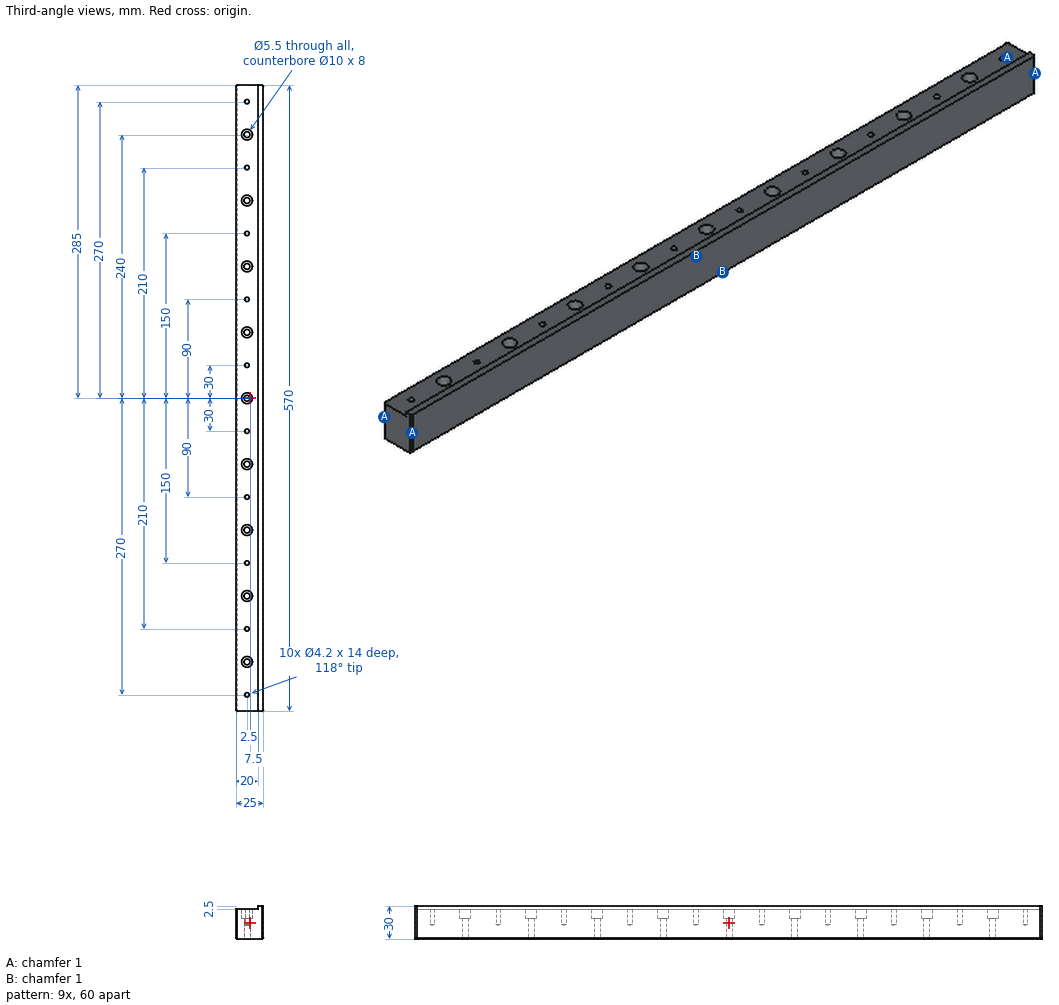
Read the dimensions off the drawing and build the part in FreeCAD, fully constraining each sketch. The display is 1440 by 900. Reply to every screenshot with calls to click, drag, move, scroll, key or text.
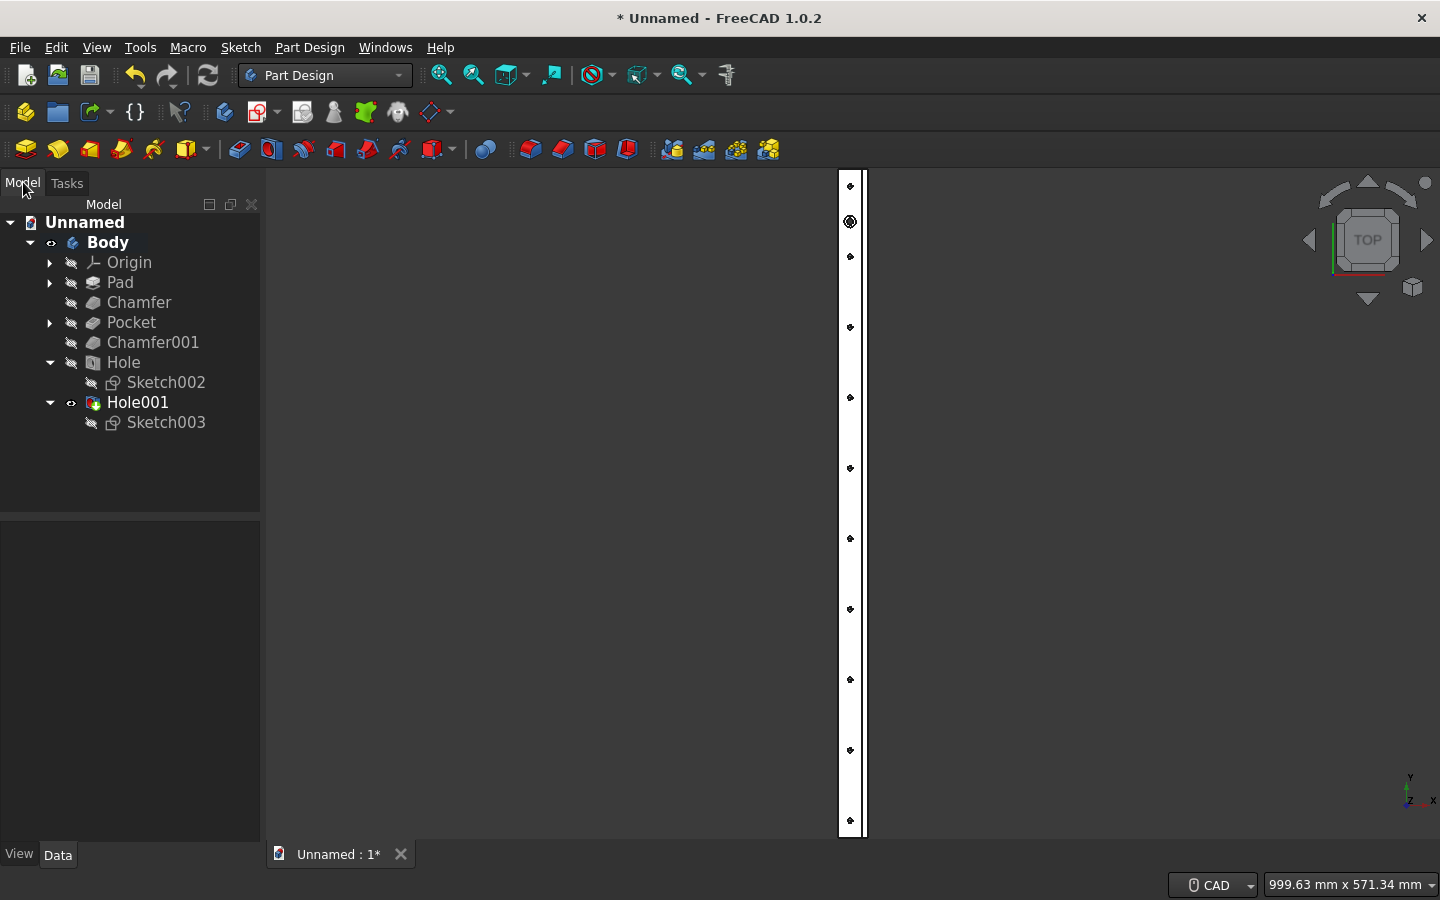
click(116, 403)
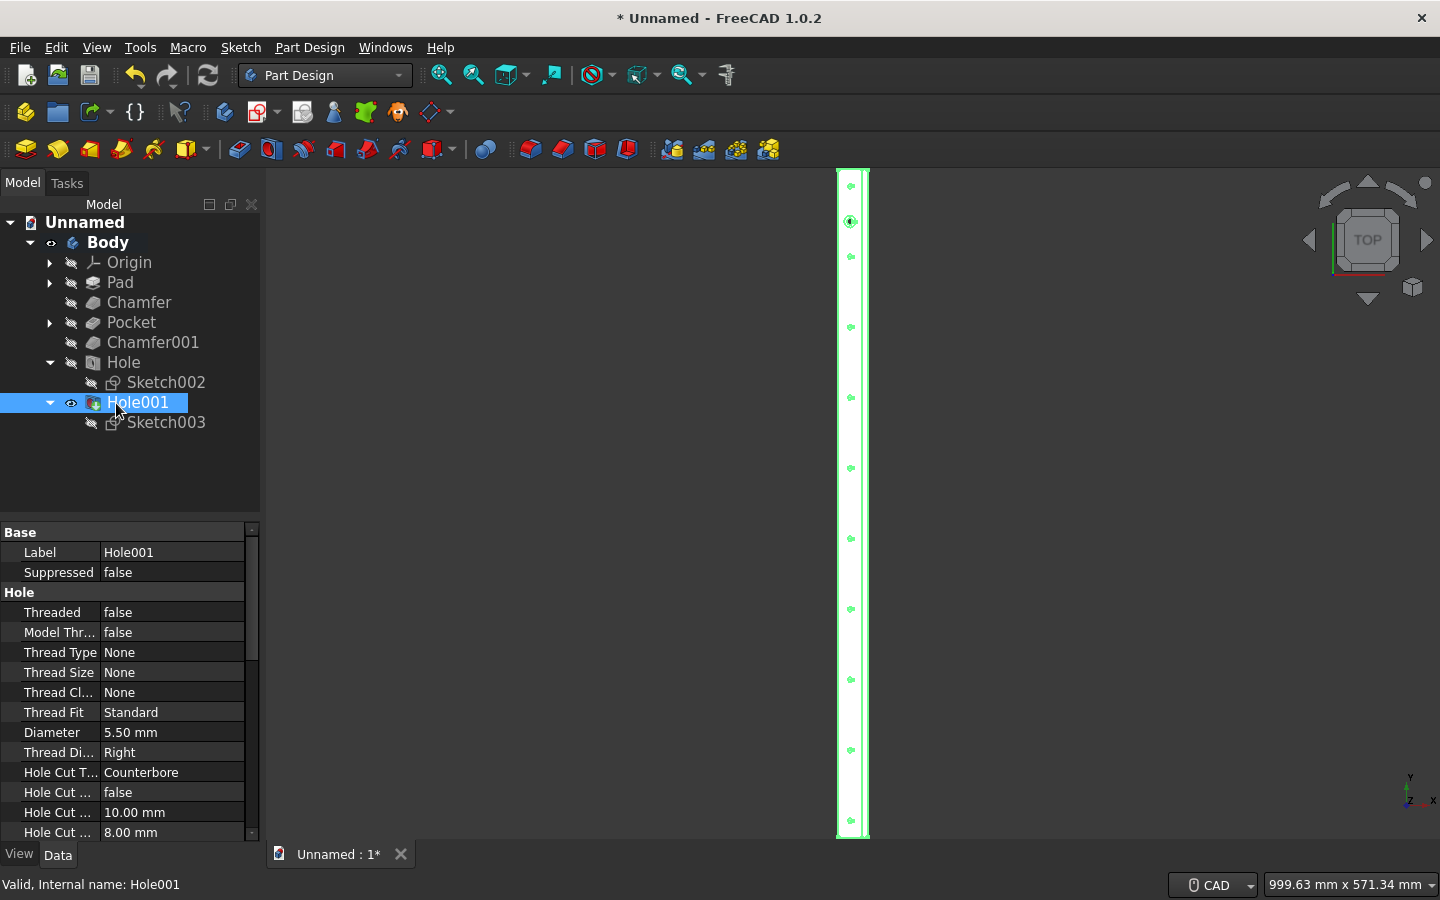
click(704, 150)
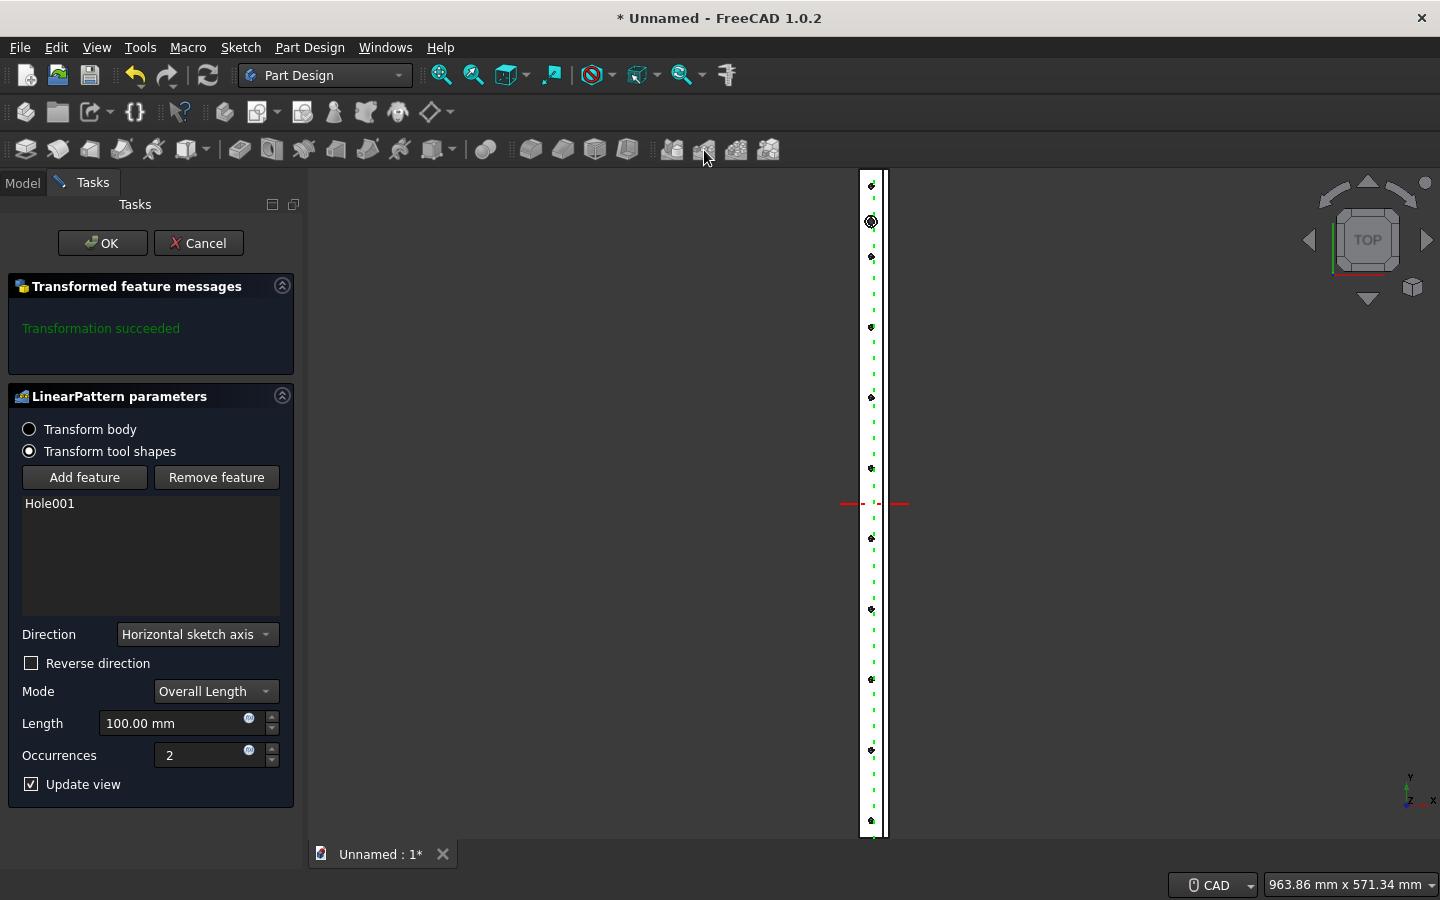
click(198, 634)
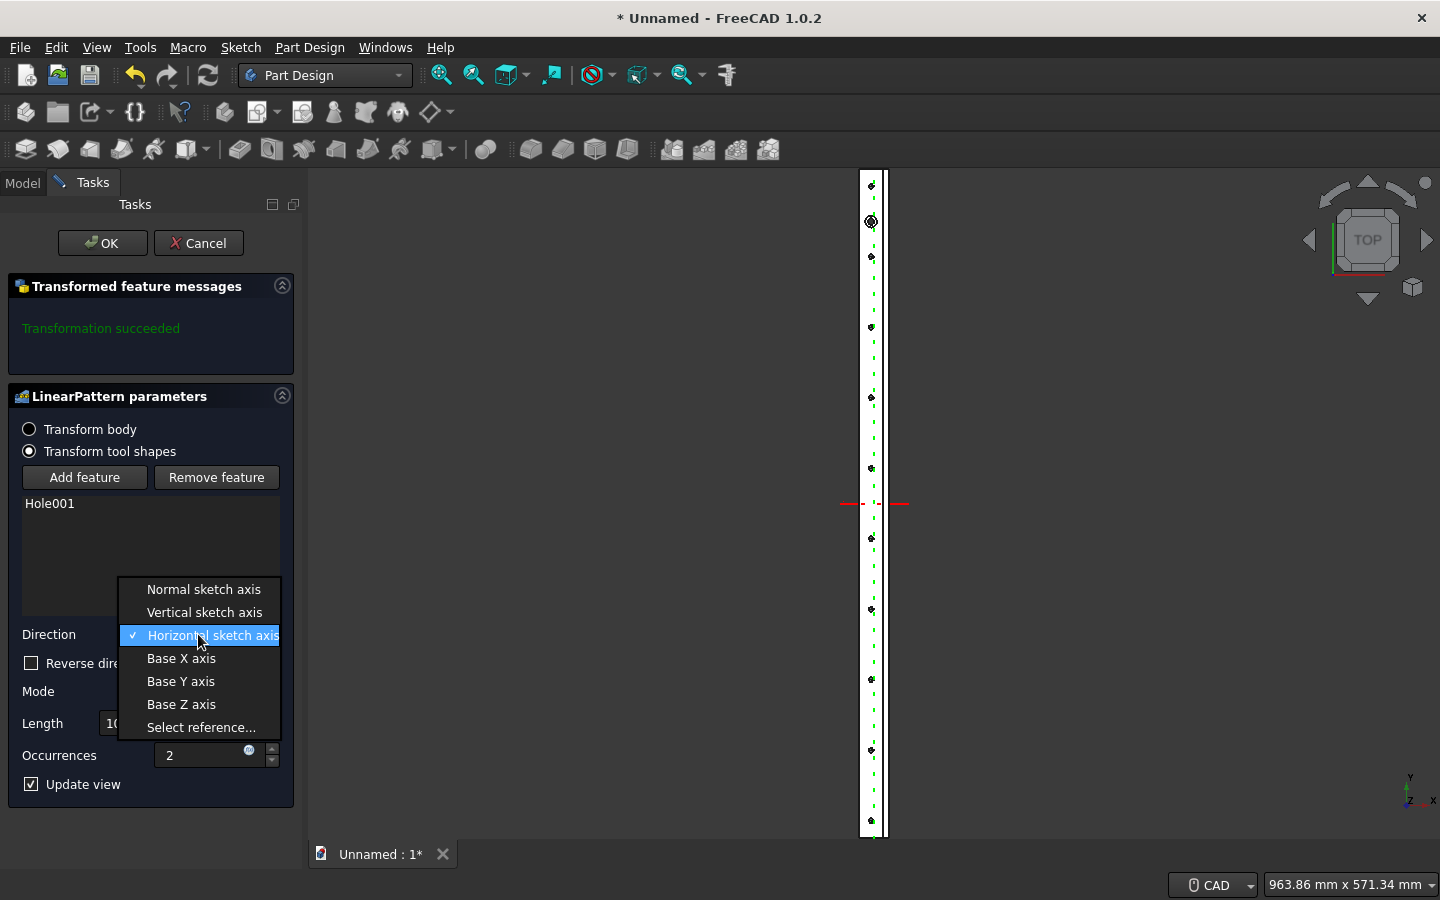
click(198, 682)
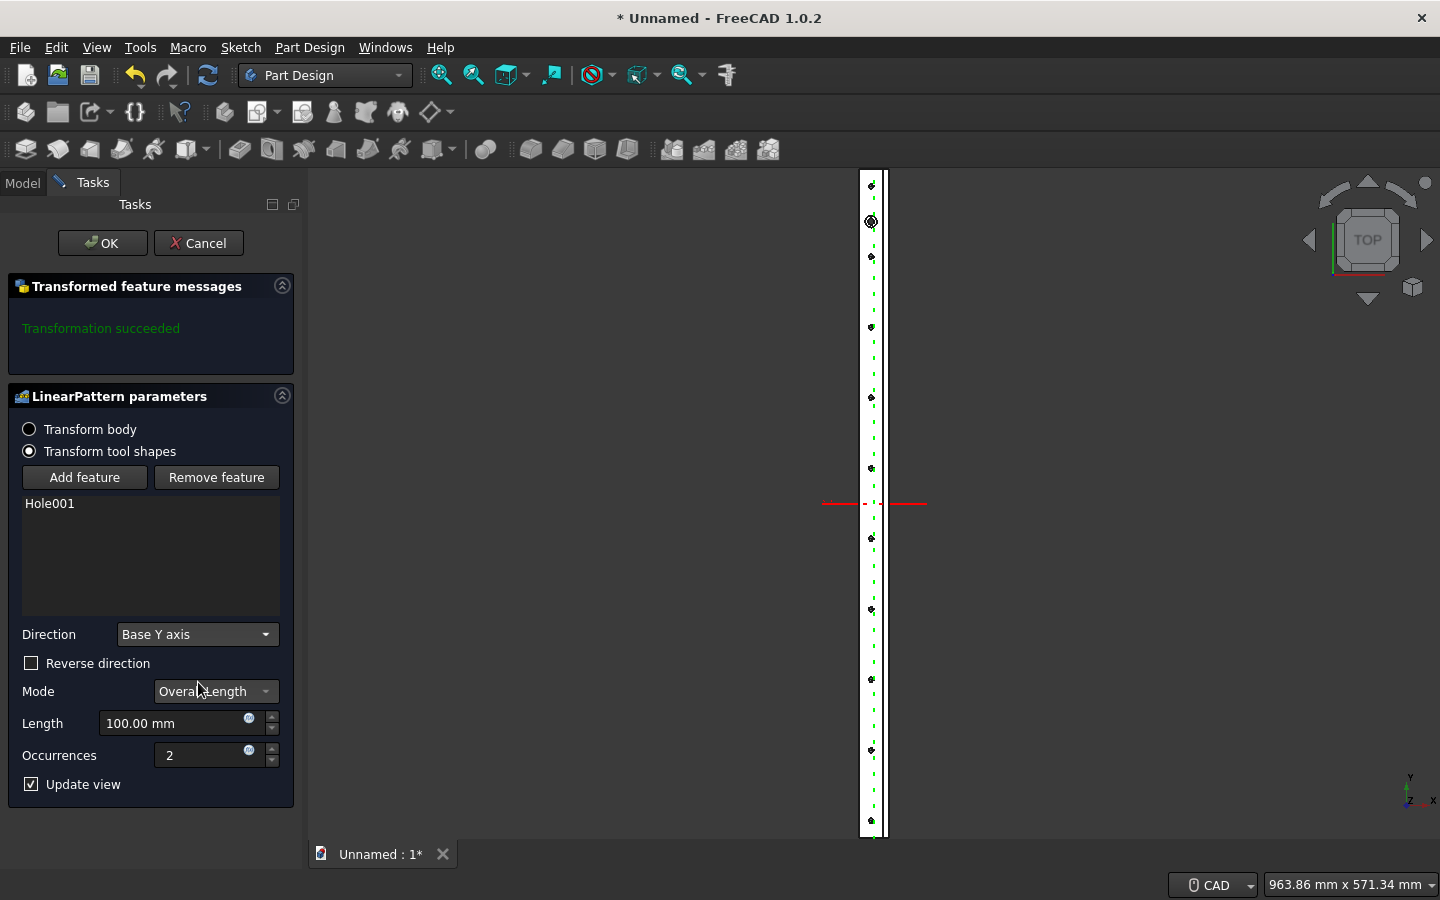
click(217, 692)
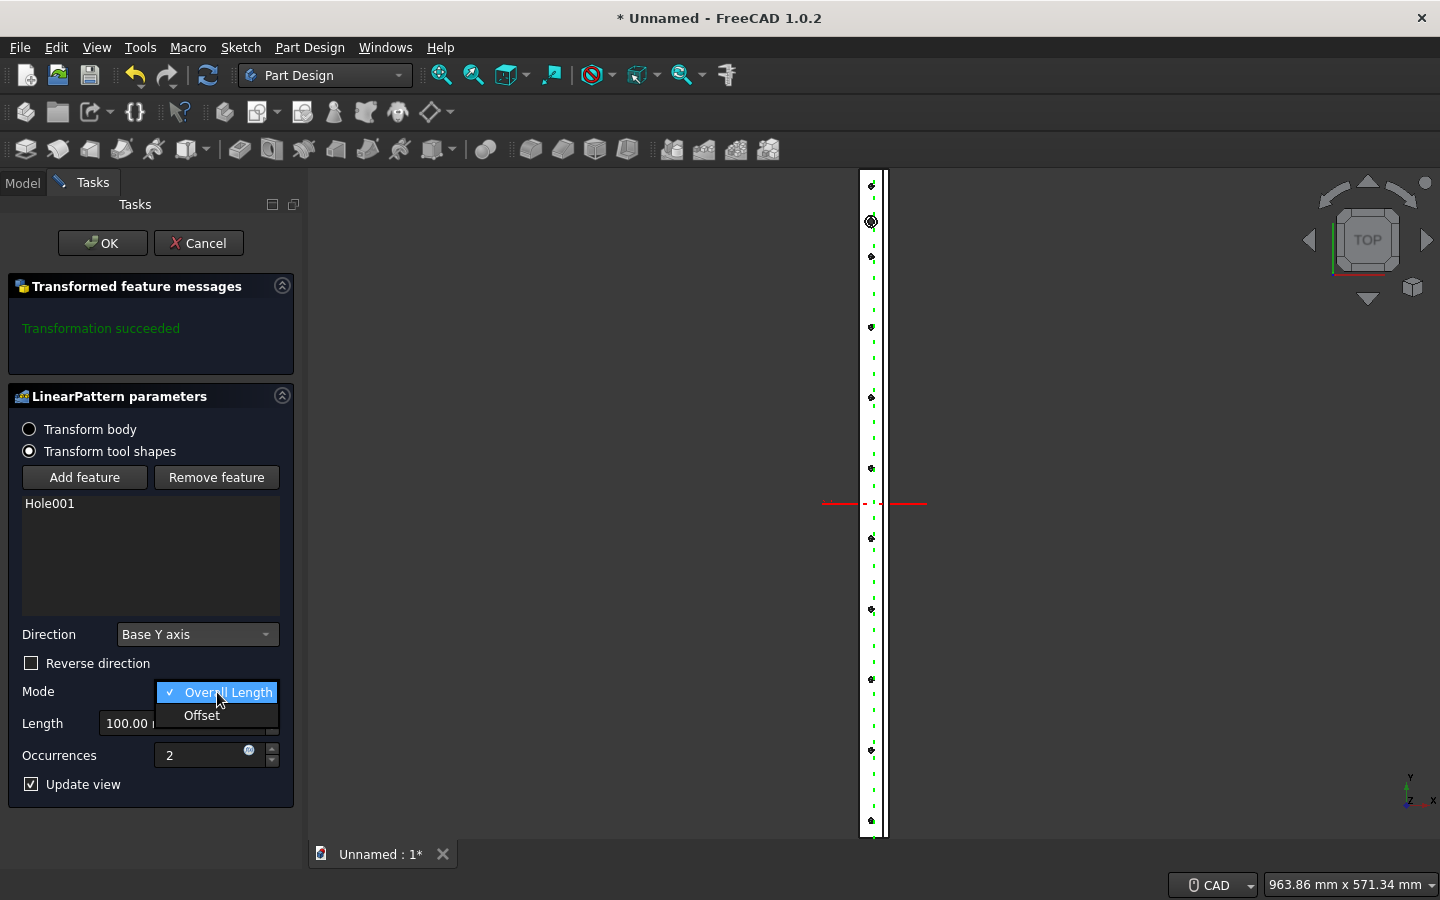
click(216, 716)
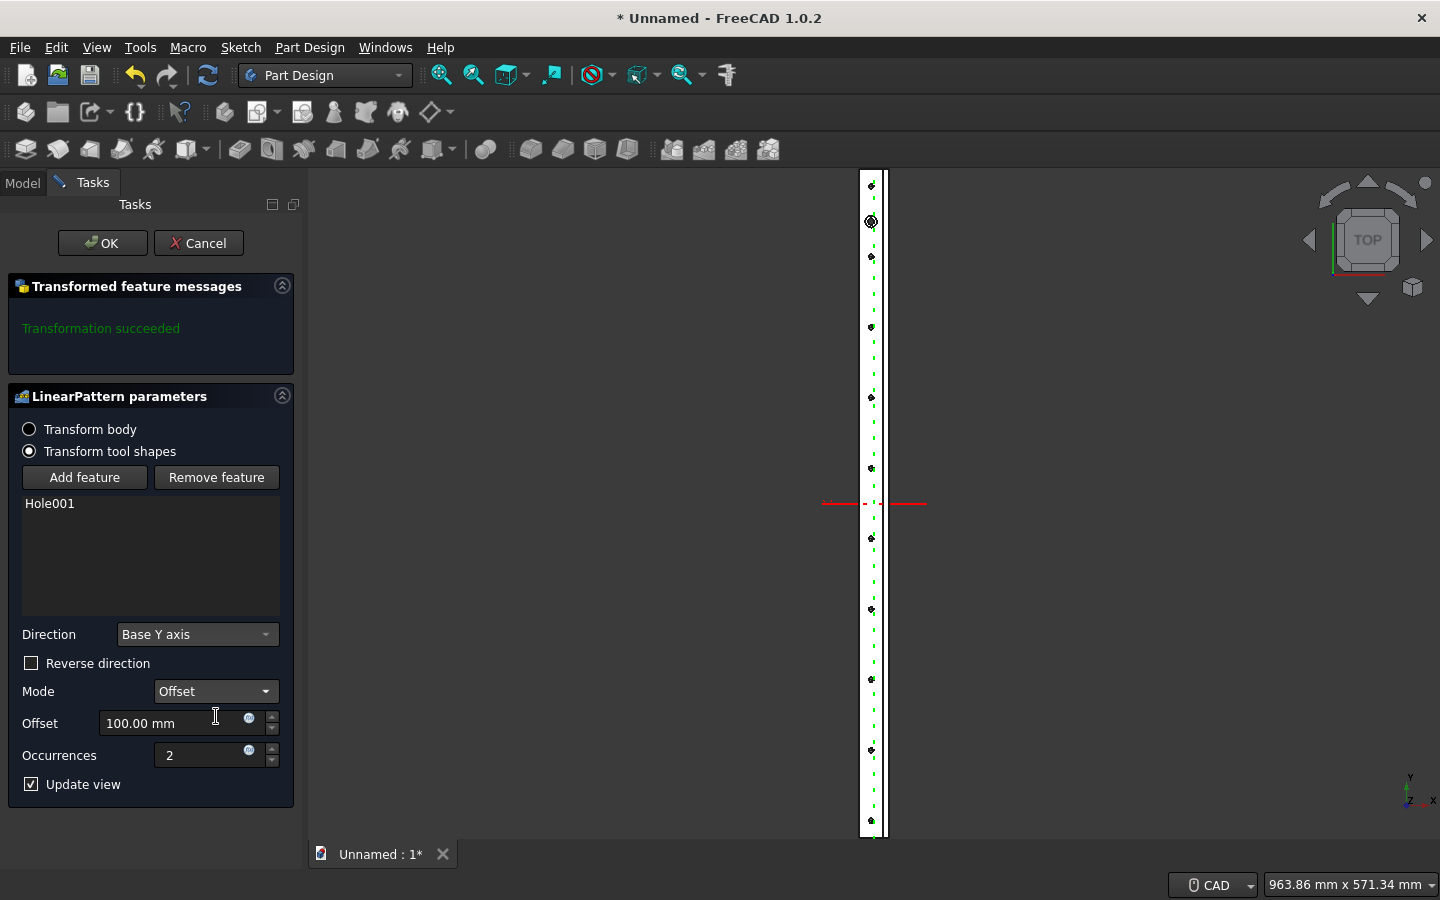
triple_click(182, 723)